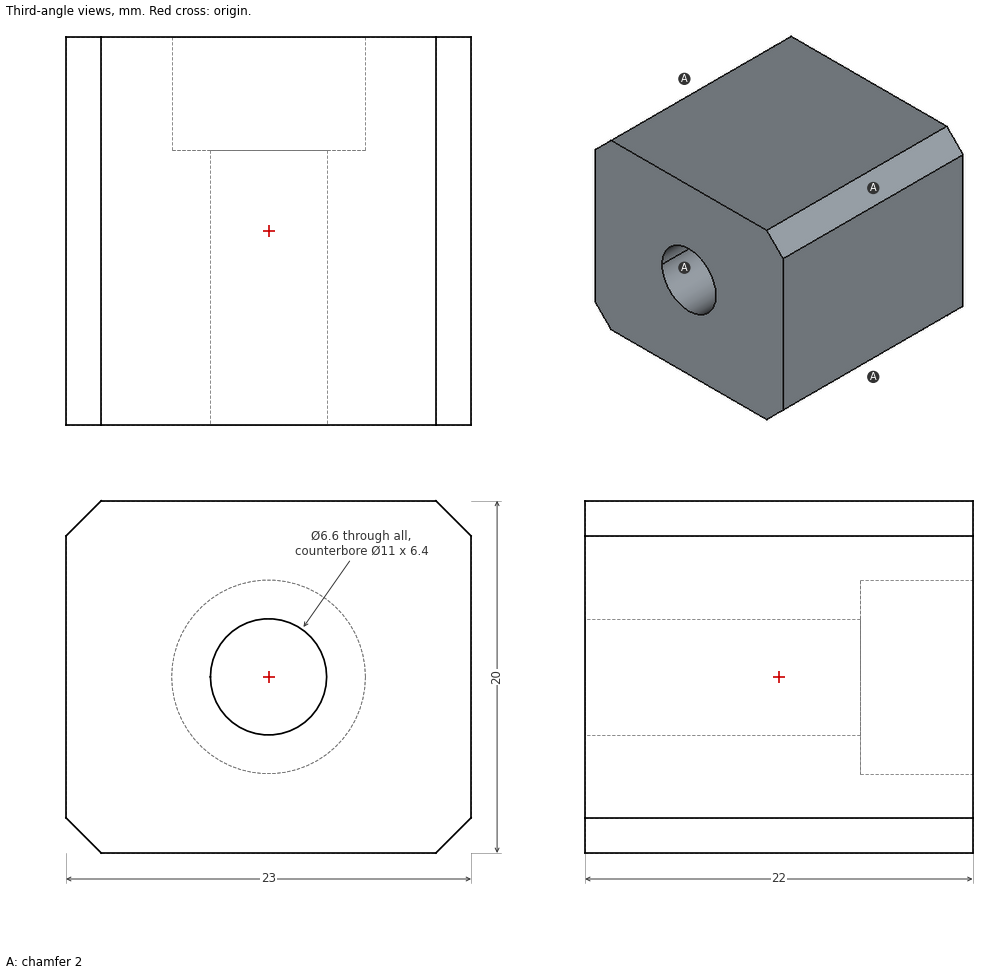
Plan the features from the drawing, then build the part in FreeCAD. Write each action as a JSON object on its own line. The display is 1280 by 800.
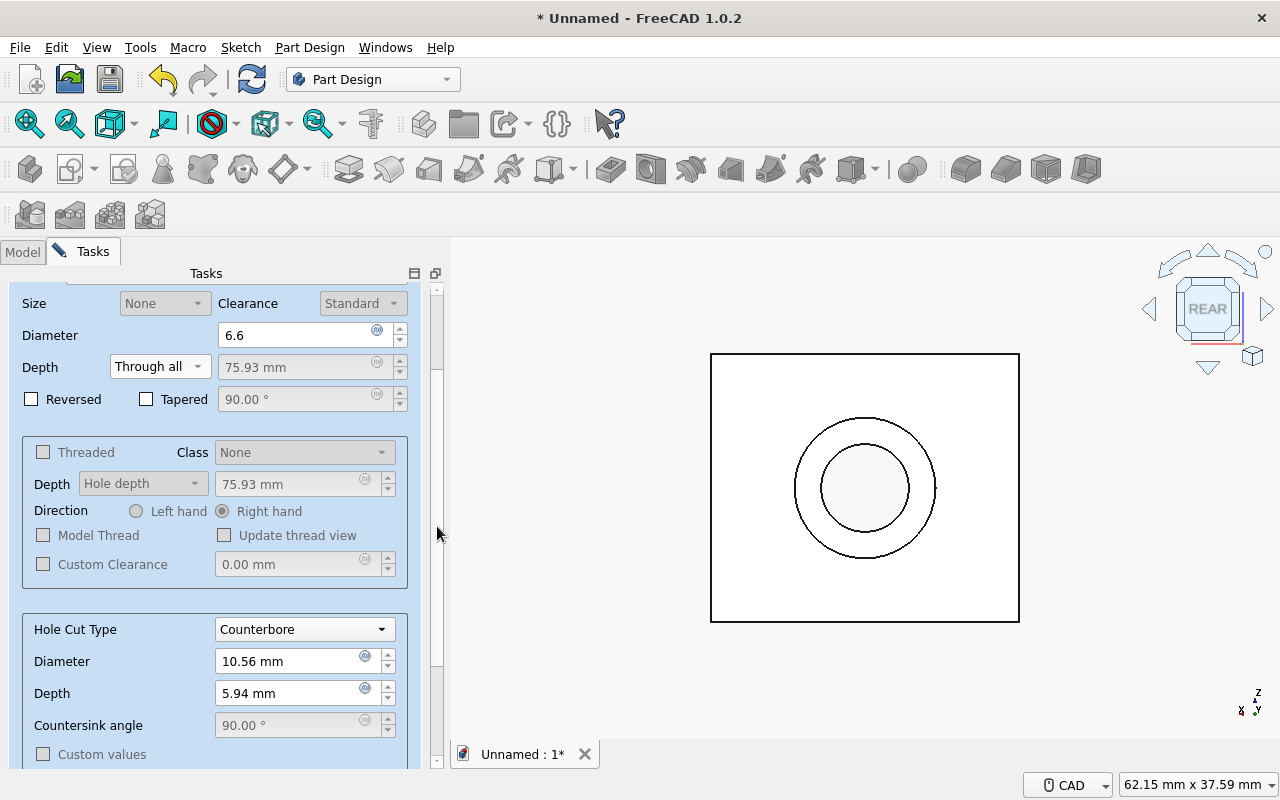
{"action": "triple_click", "coordinate": [298, 661]}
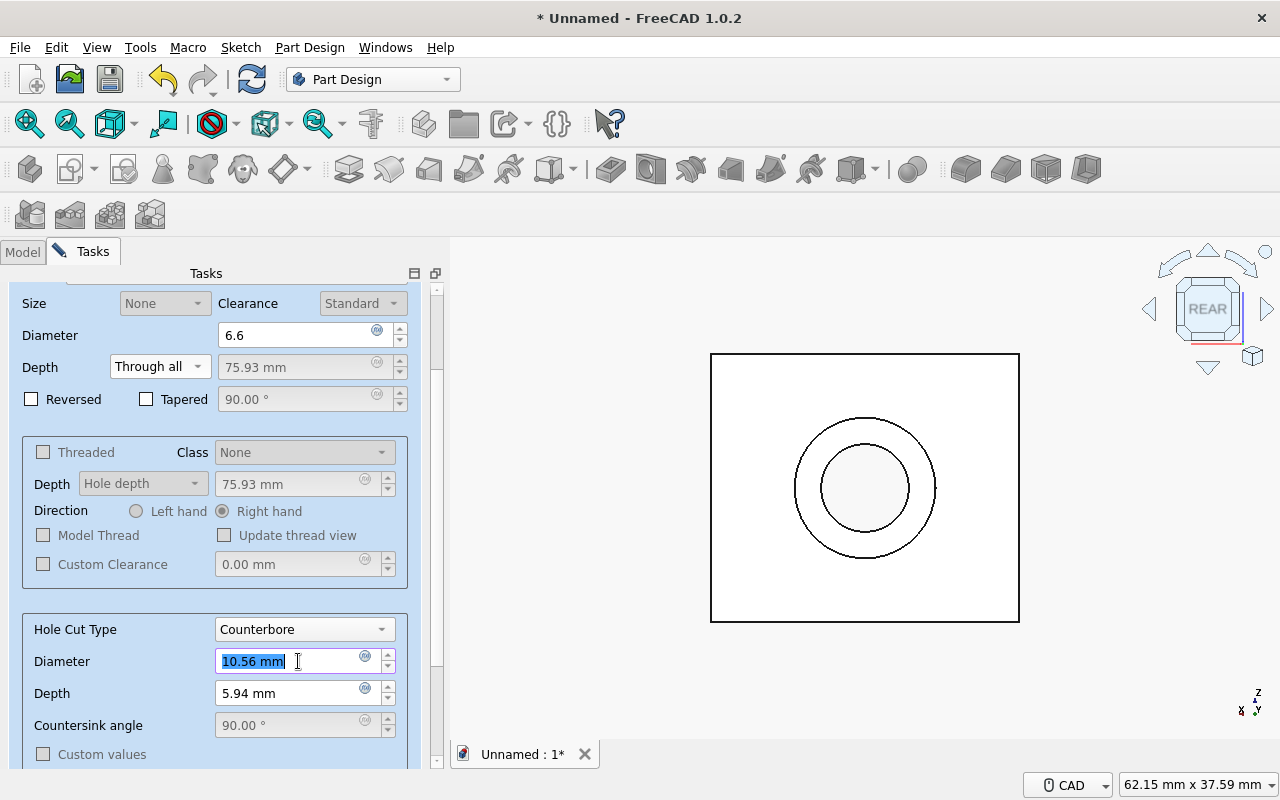
{"action": "type", "text": "11"}
{"action": "key", "text": "Tab"}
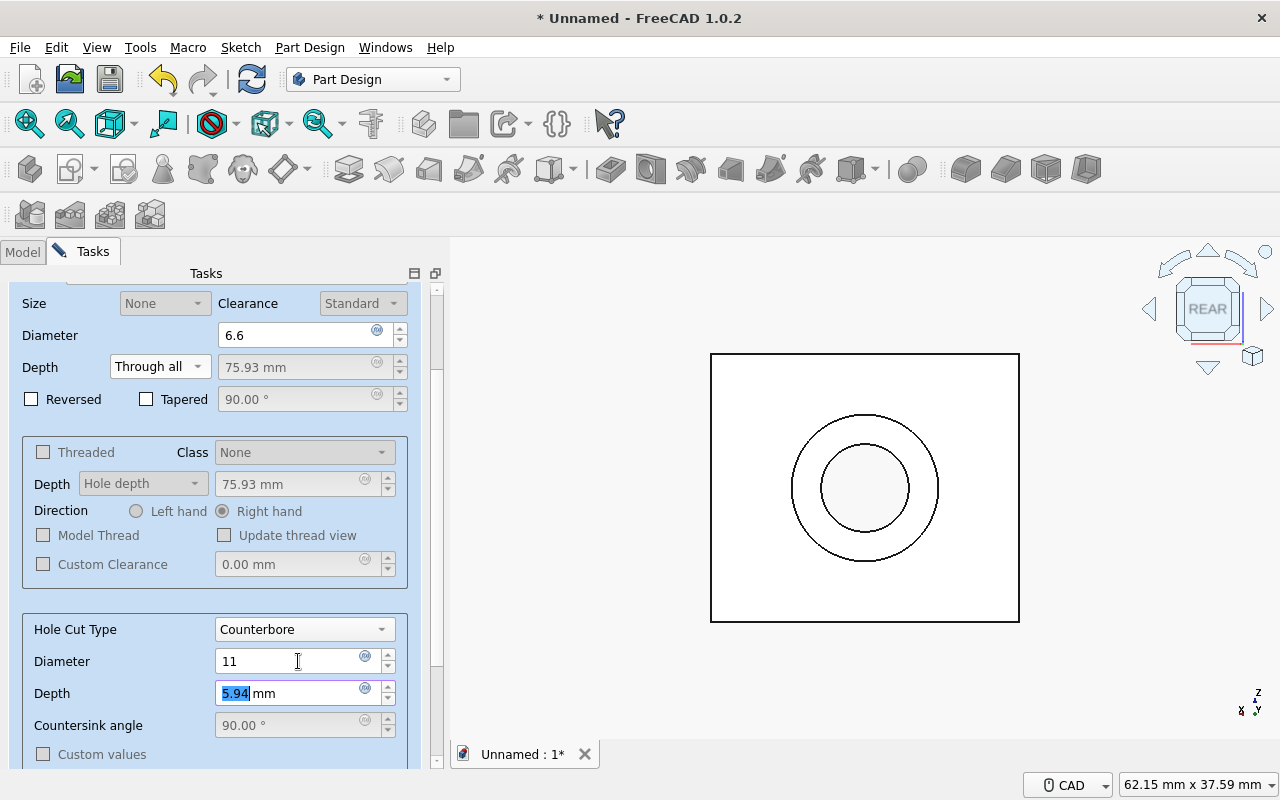
{"action": "type", "text": "6.4"}
{"action": "key", "text": "Tab"}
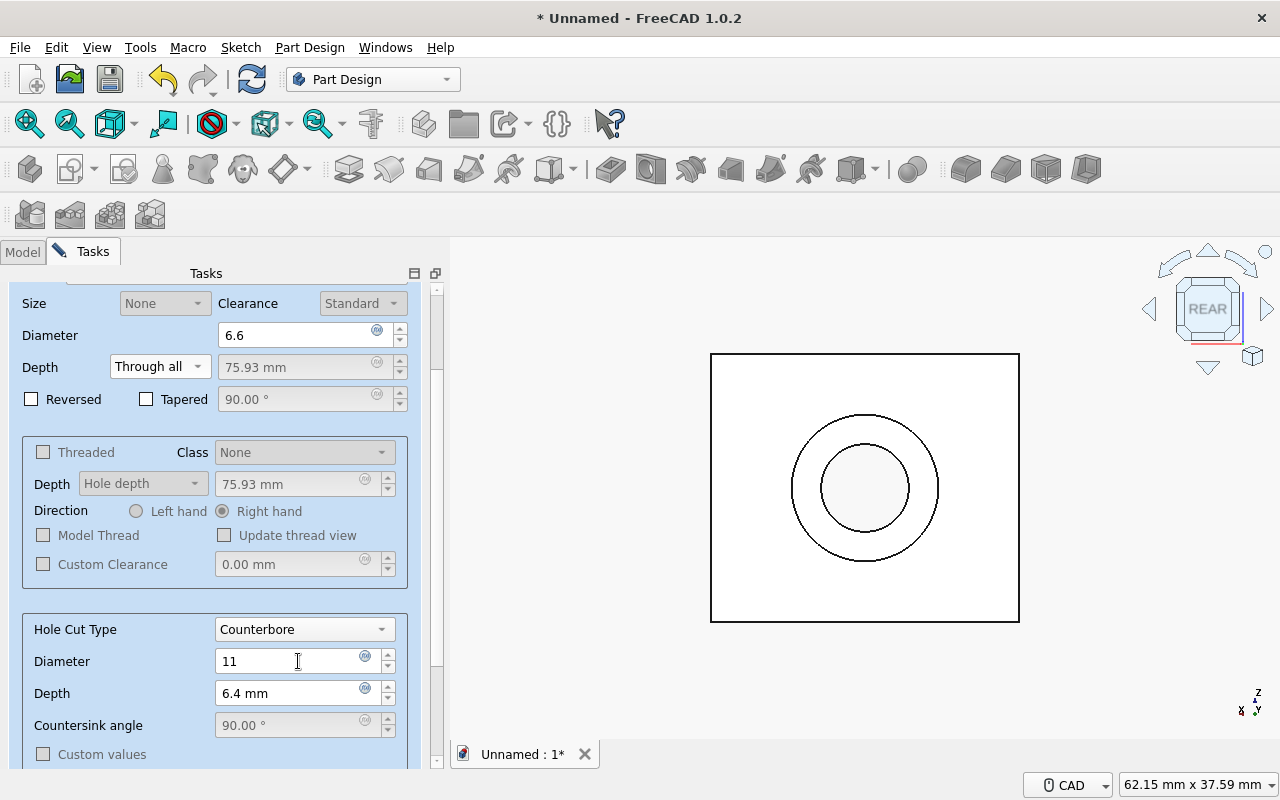
{"action": "scroll", "coordinate": [437, 526], "scroll_direction": "up", "scroll_amount": 3}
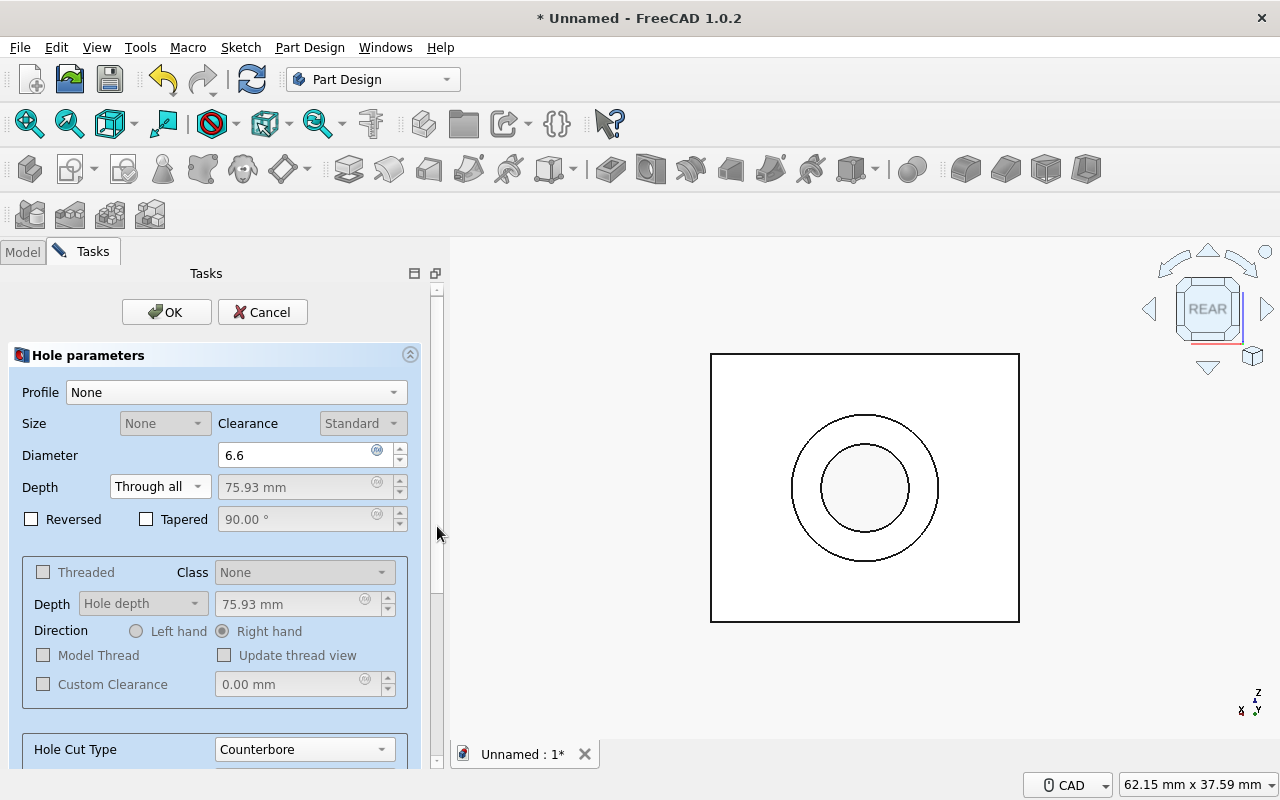
{"action": "left_click", "coordinate": [167, 312]}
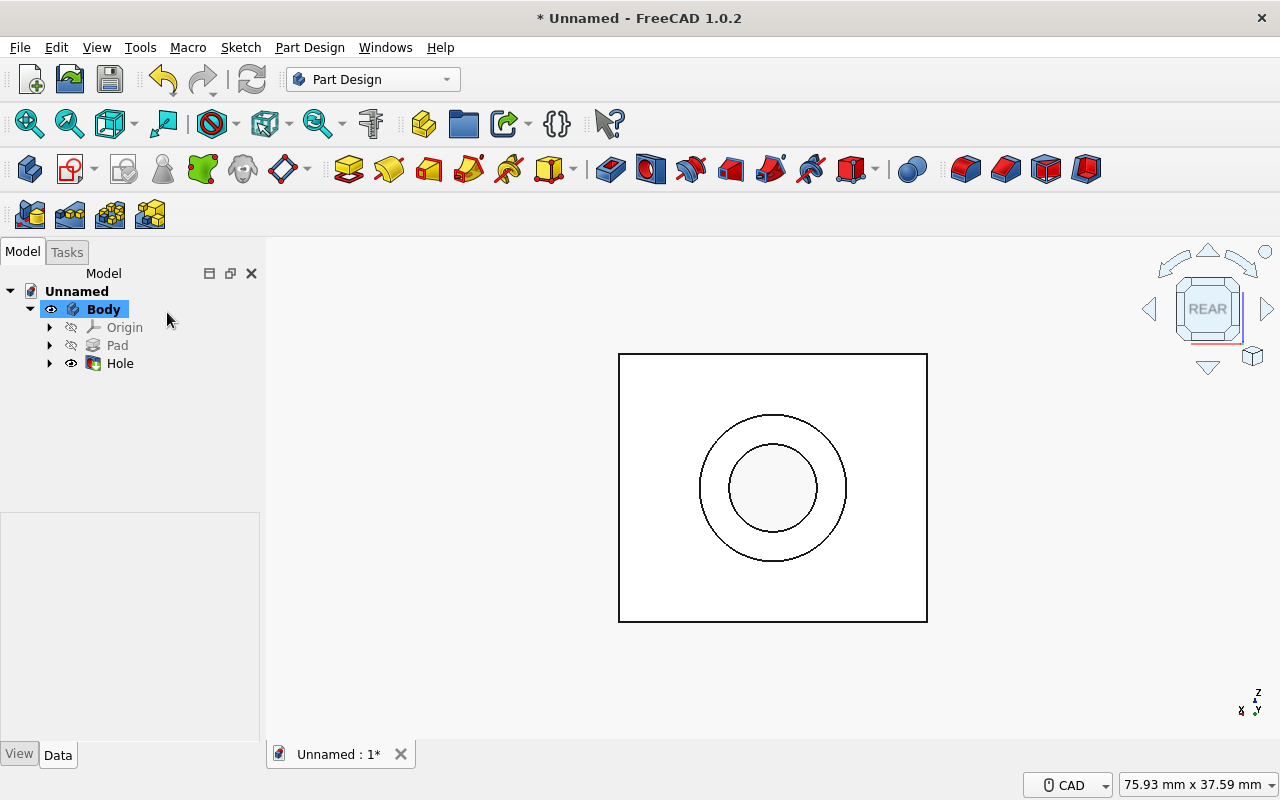
{"action": "key", "text": "0"}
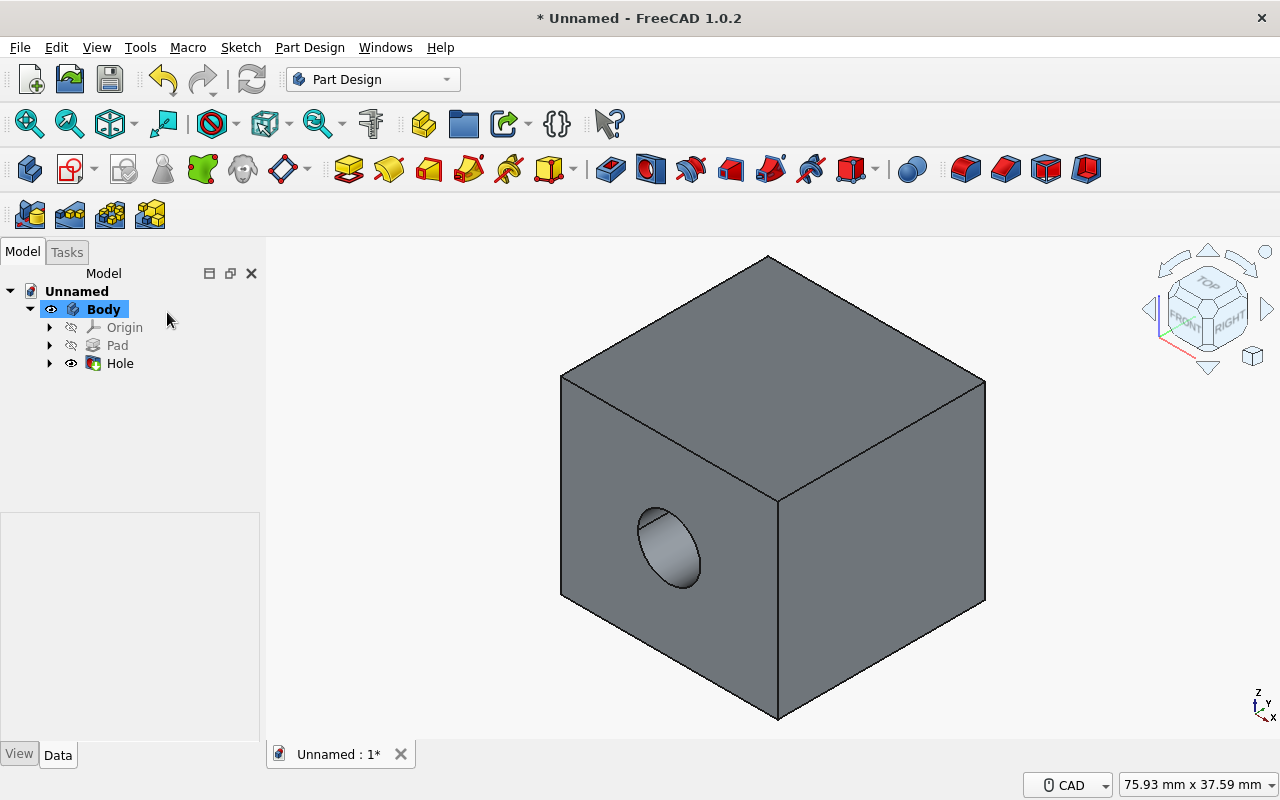
{"action": "left_click", "coordinate": [882, 441]}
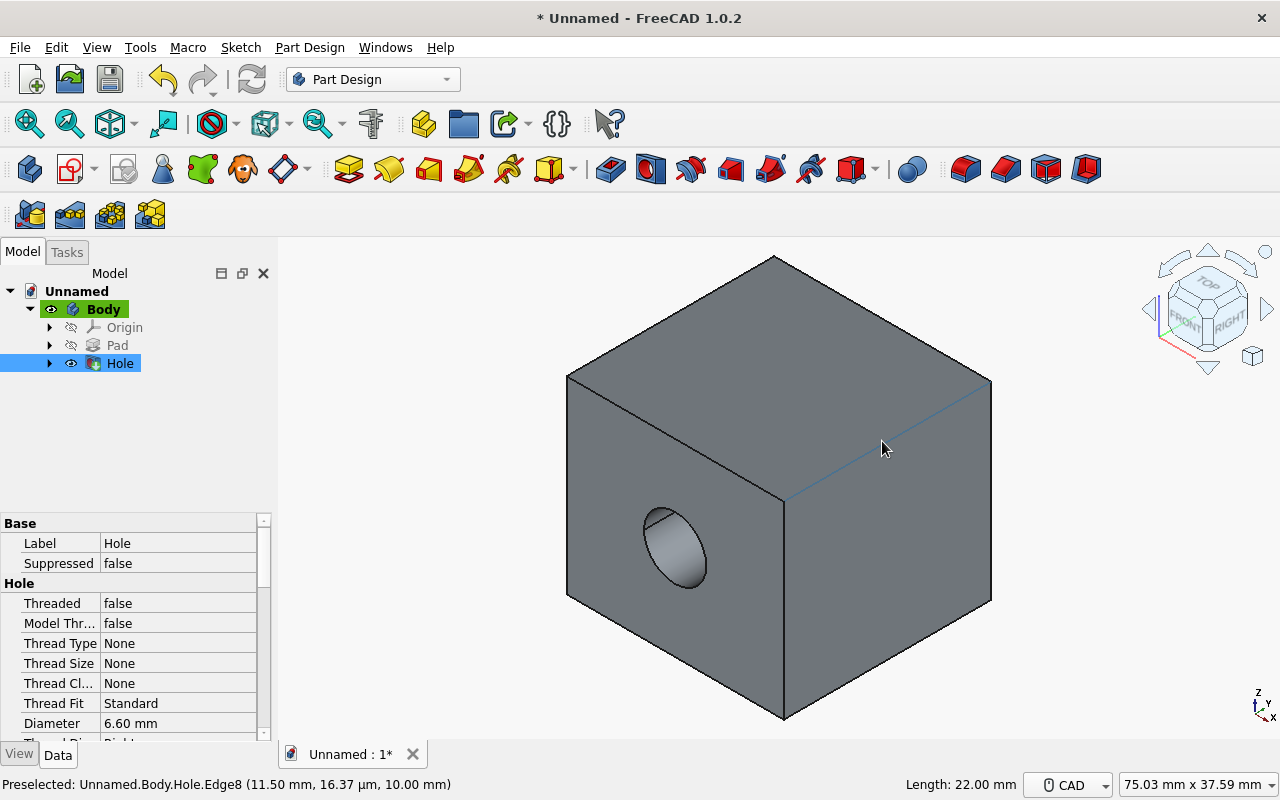
{"action": "key", "text": "2"}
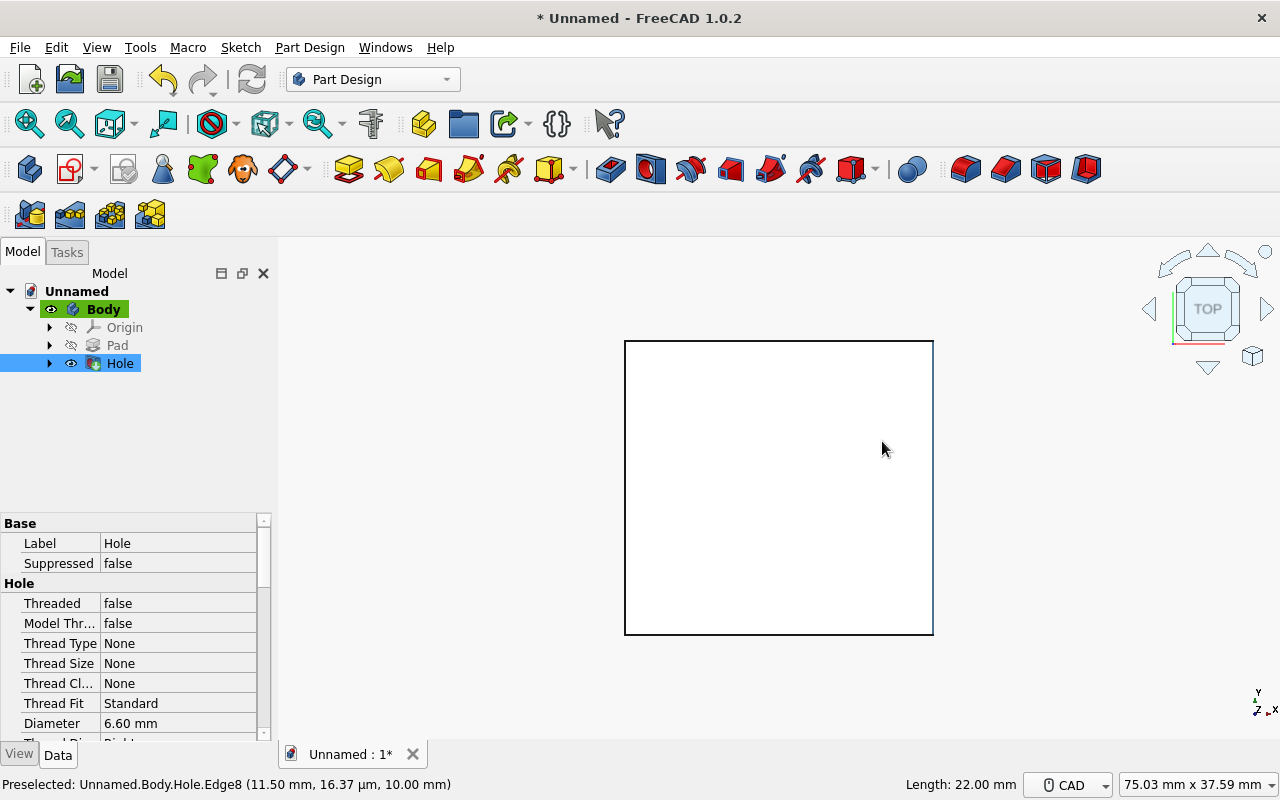
{"action": "left_click", "coordinate": [625, 487], "text": "ctrl"}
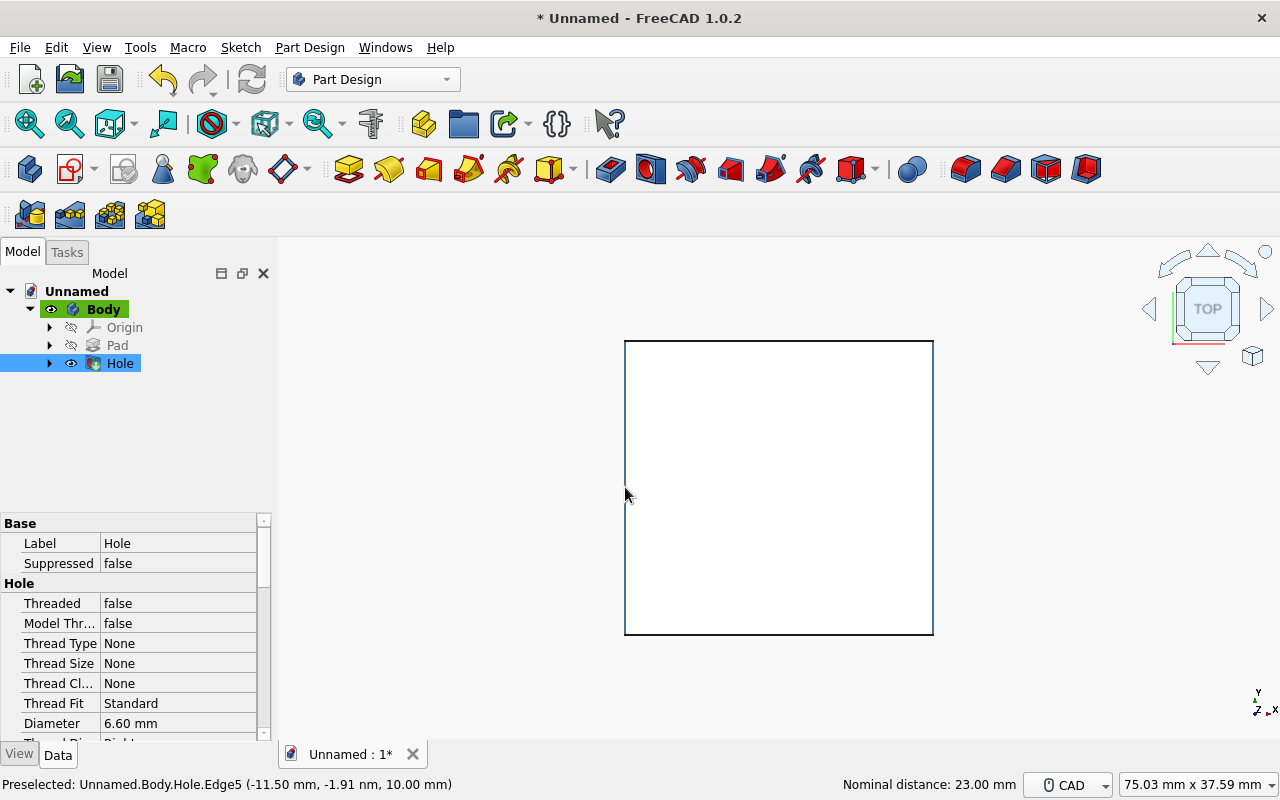
{"action": "key", "text": "1"}